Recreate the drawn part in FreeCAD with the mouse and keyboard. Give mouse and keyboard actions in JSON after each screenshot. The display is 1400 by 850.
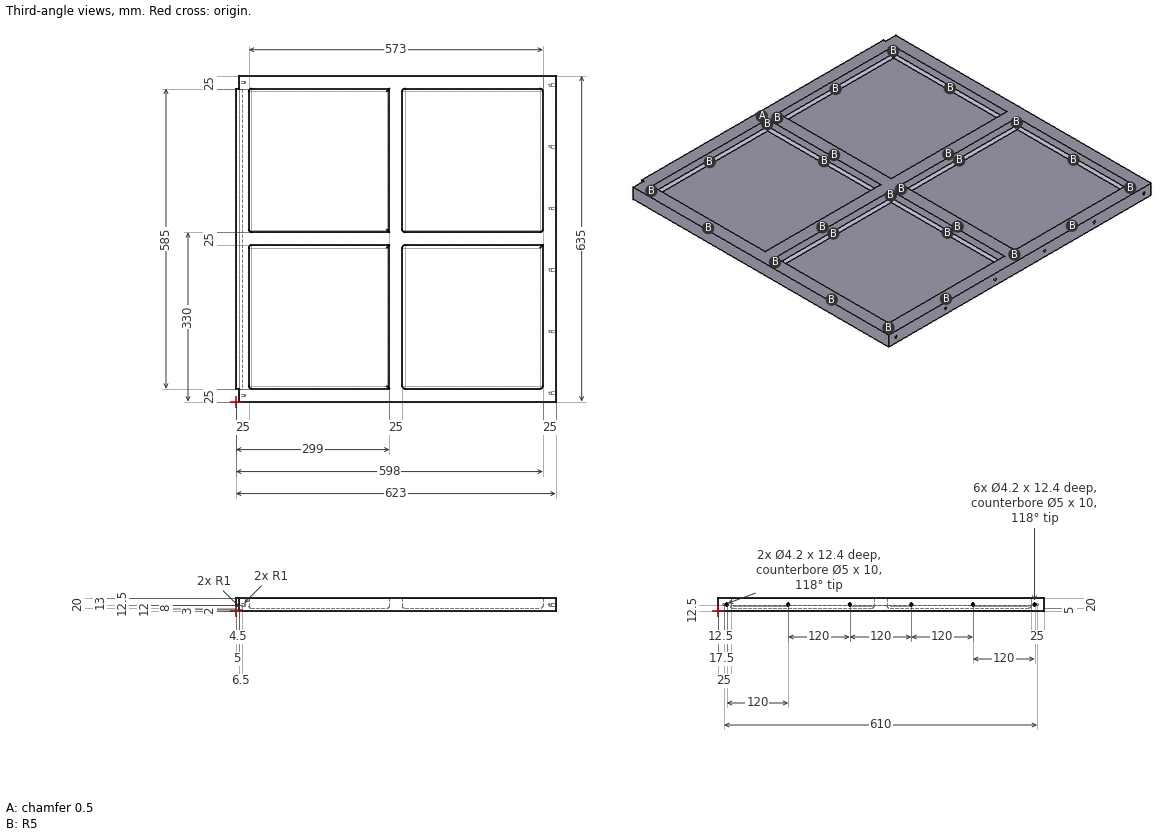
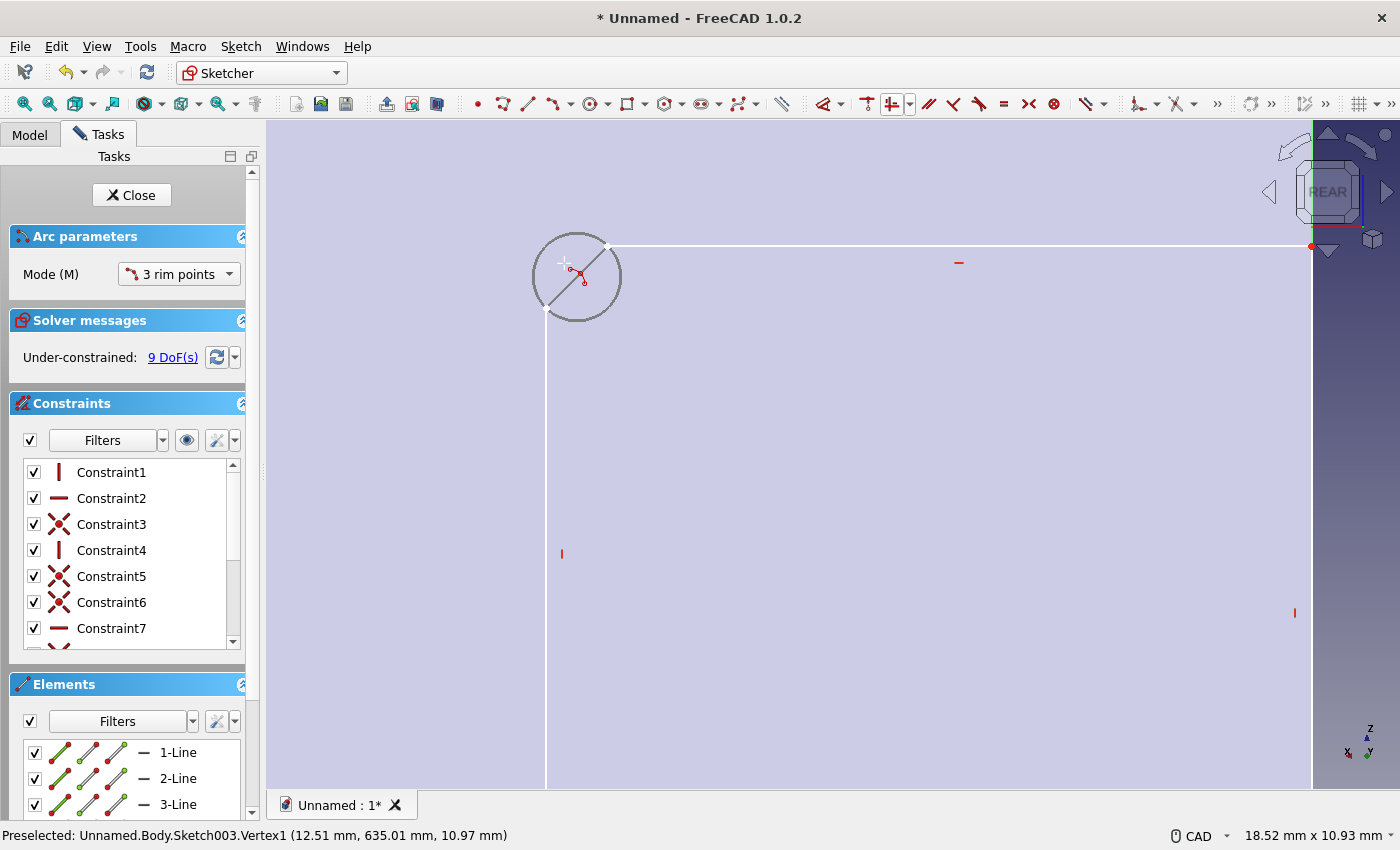
{"action": "left_click", "coordinate": [564, 263]}
{"action": "key", "text": "Escape"}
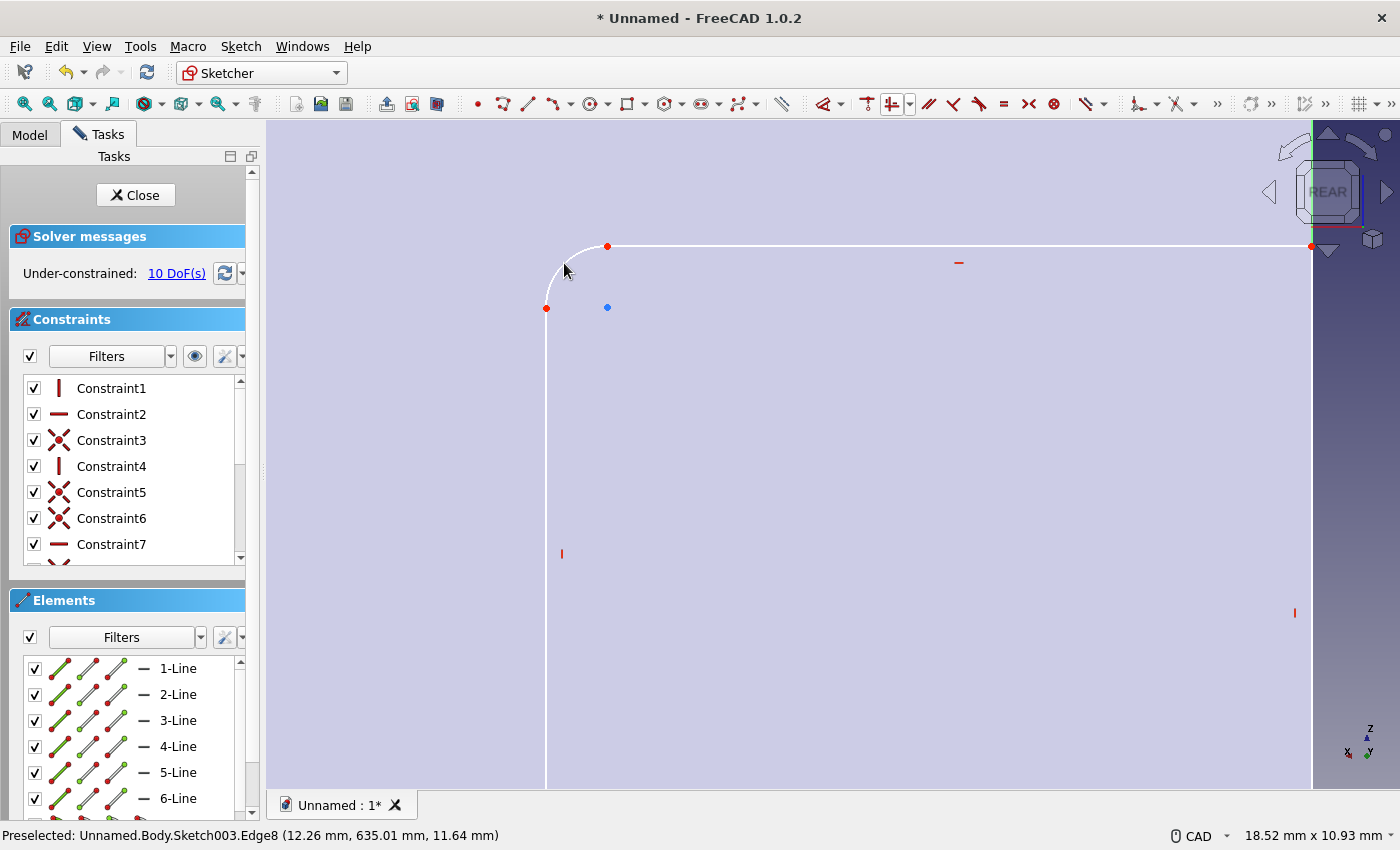
{"action": "left_click", "coordinate": [546, 455]}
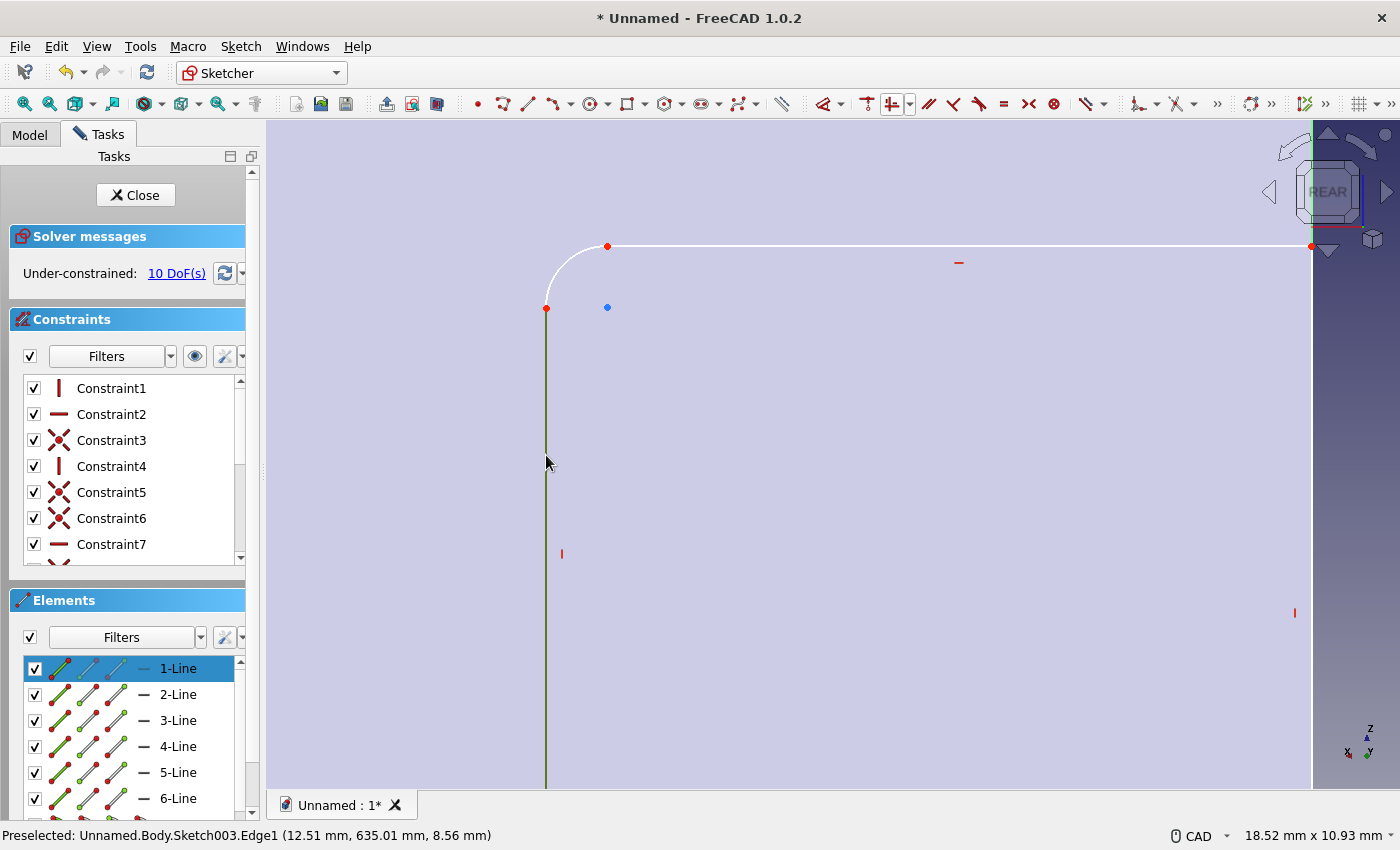
{"action": "scroll", "coordinate": [564, 262], "scroll_direction": "down", "scroll_amount": 3}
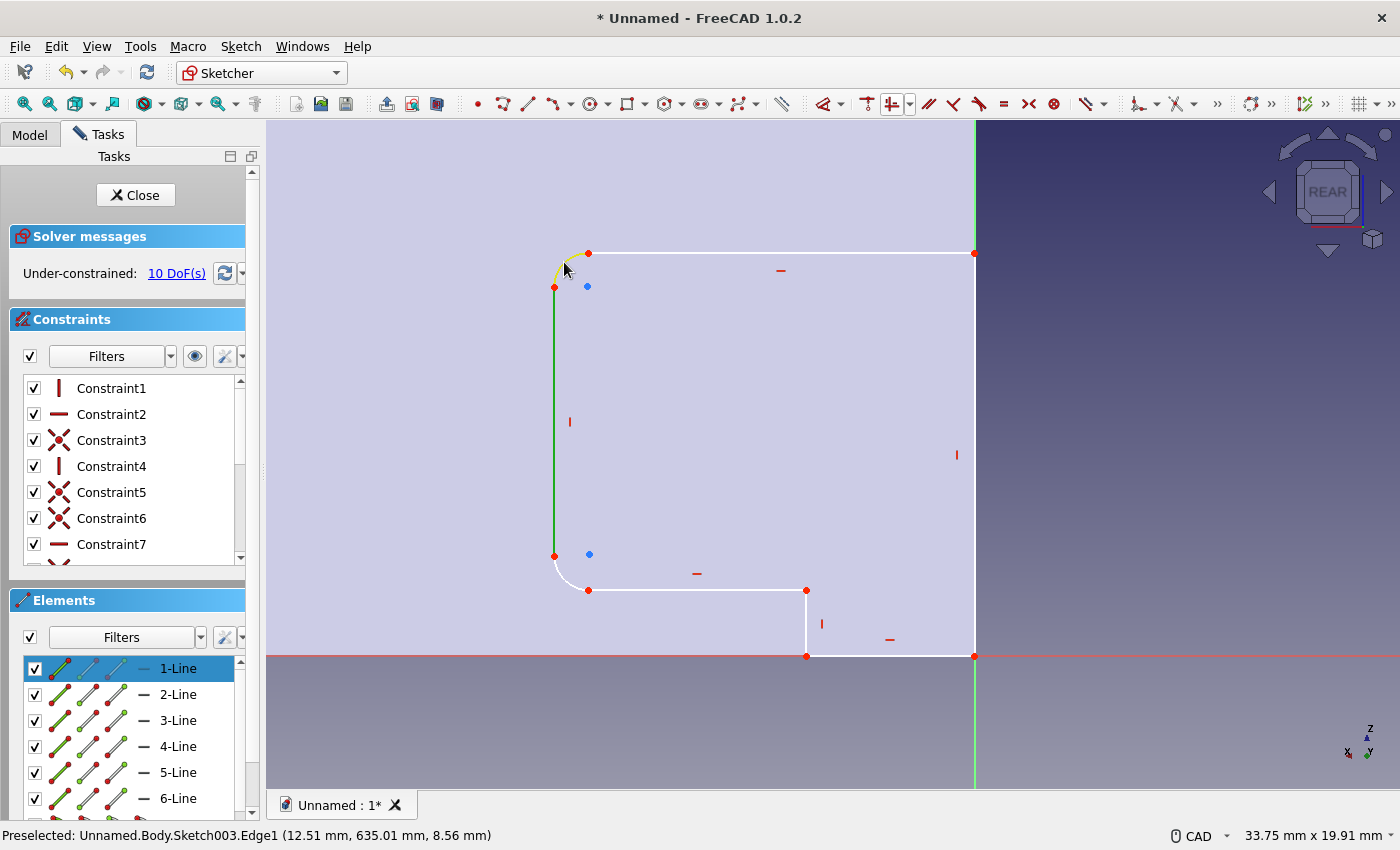
{"action": "left_click", "coordinate": [558, 572]}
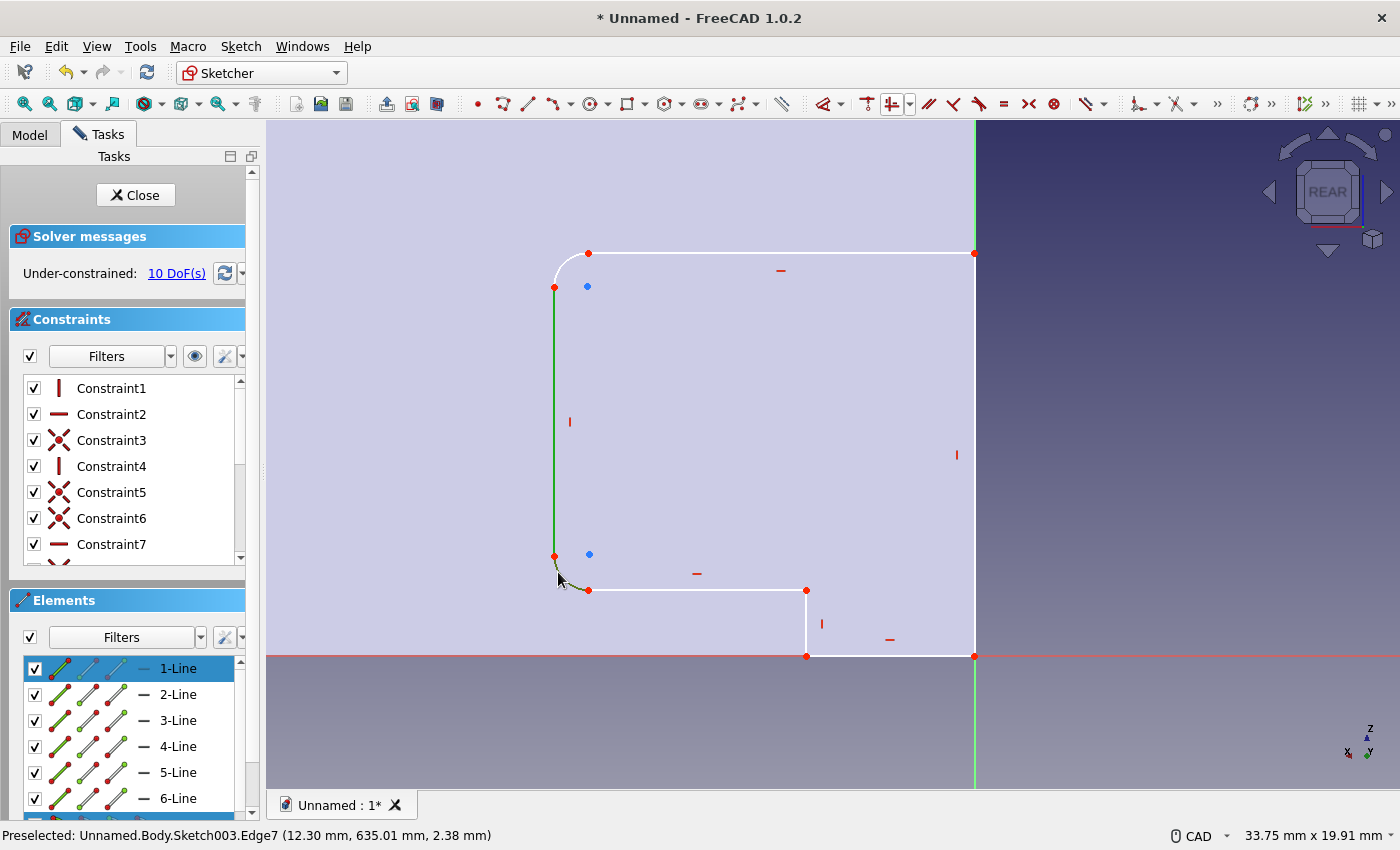
{"action": "left_click", "coordinate": [979, 104]}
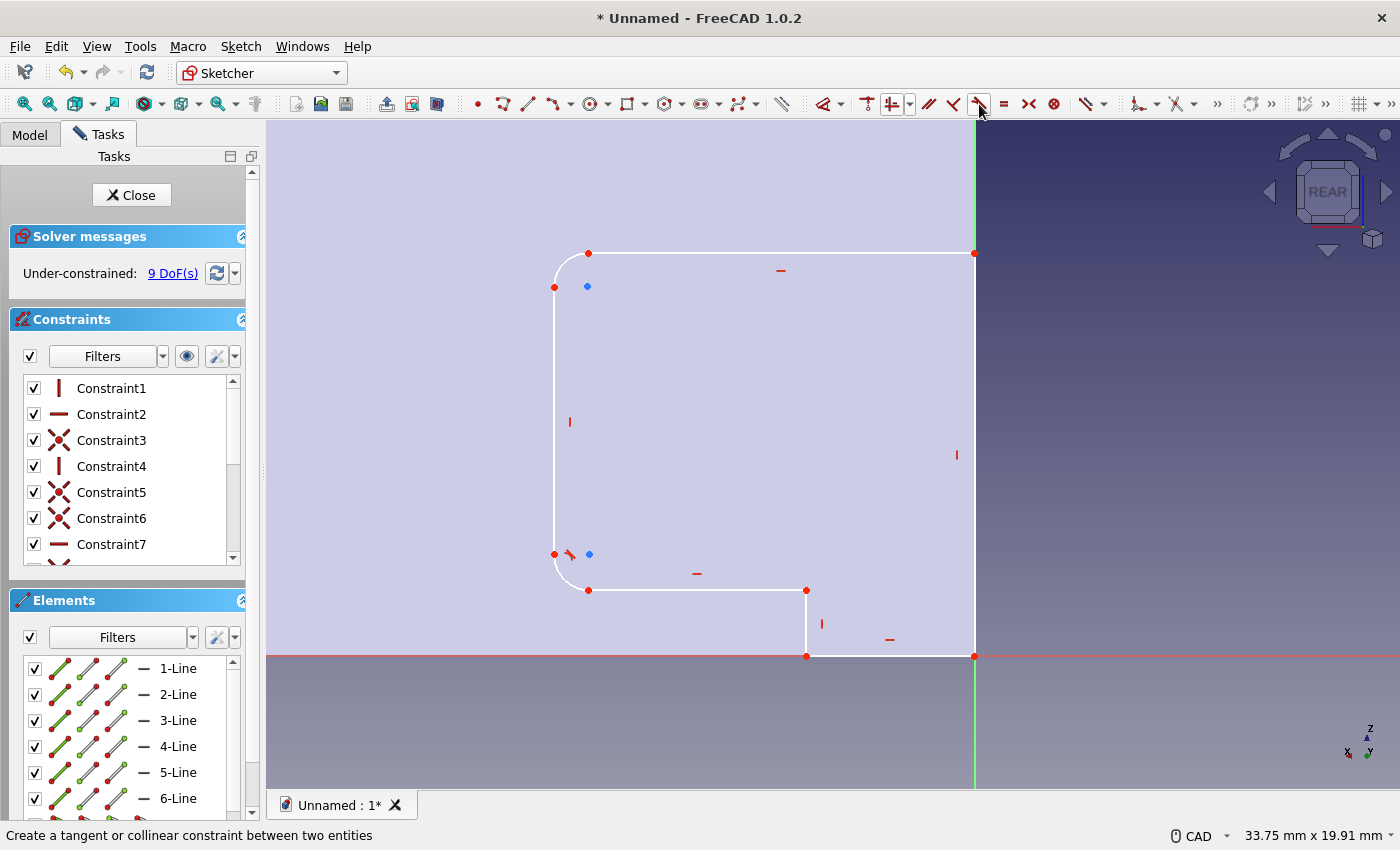
{"action": "left_click", "coordinate": [554, 368]}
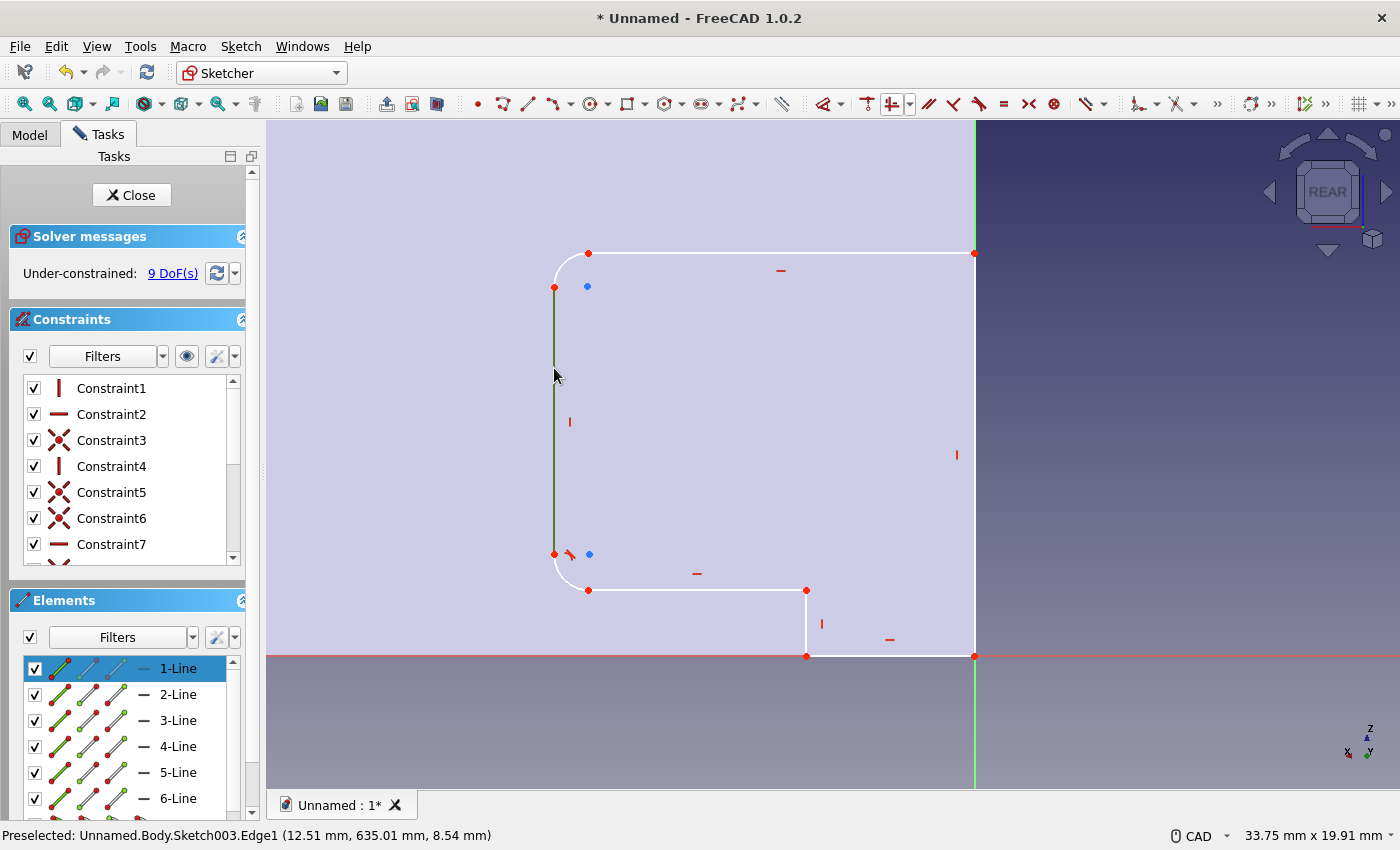
{"action": "left_click", "coordinate": [573, 257]}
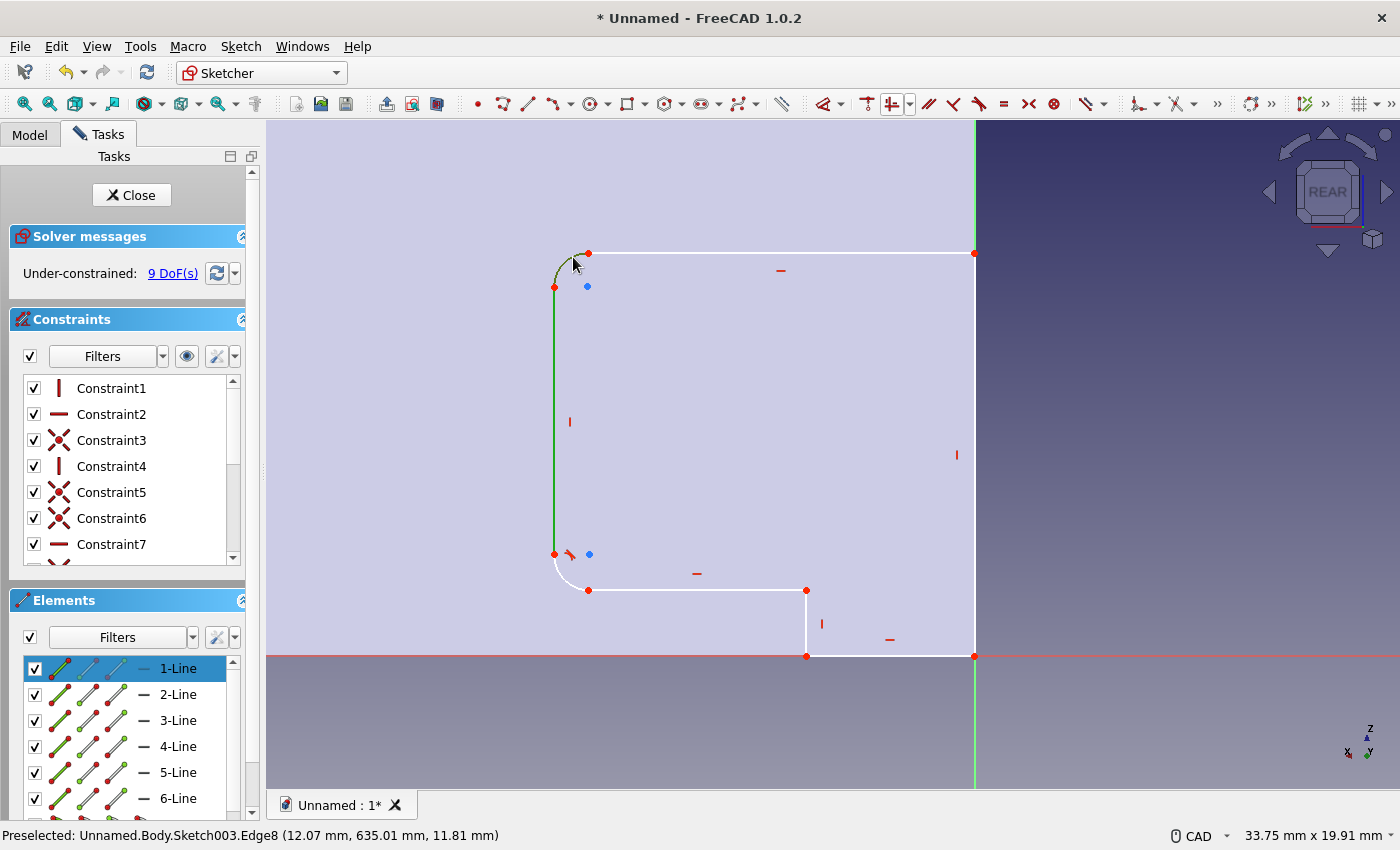
{"action": "left_click", "coordinate": [979, 104]}